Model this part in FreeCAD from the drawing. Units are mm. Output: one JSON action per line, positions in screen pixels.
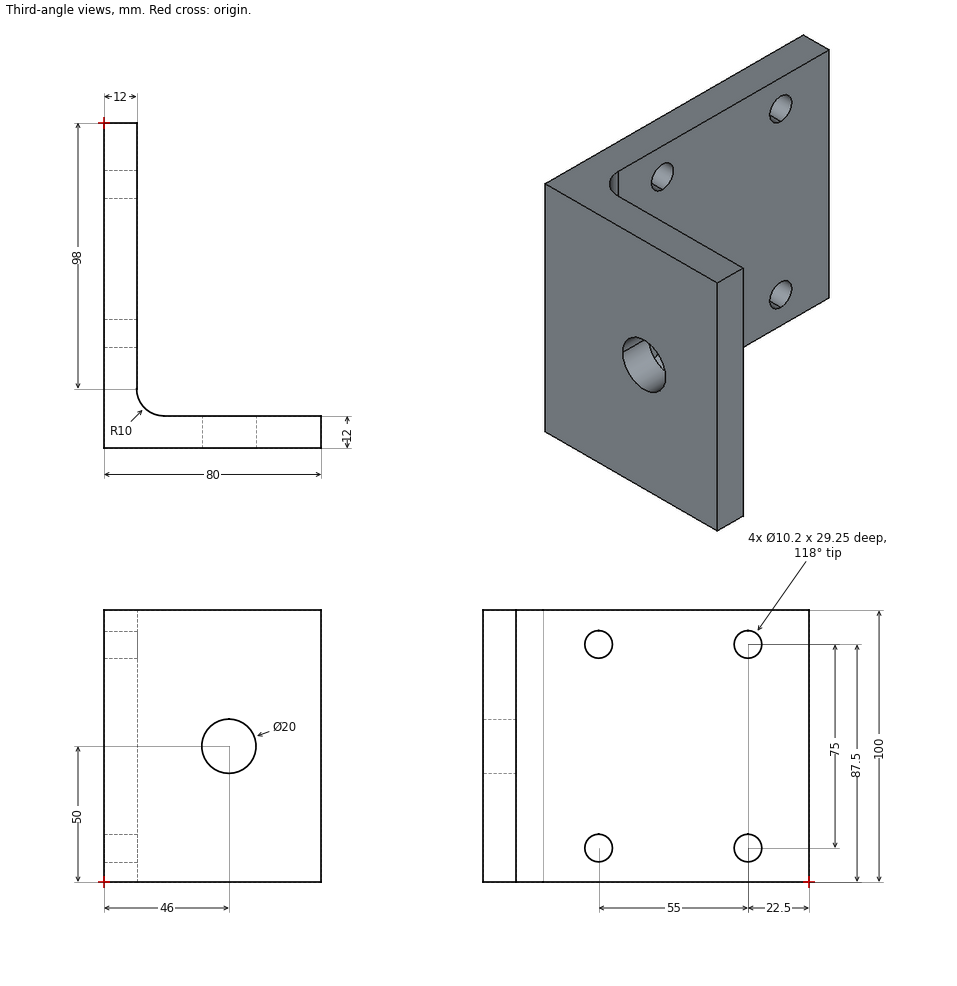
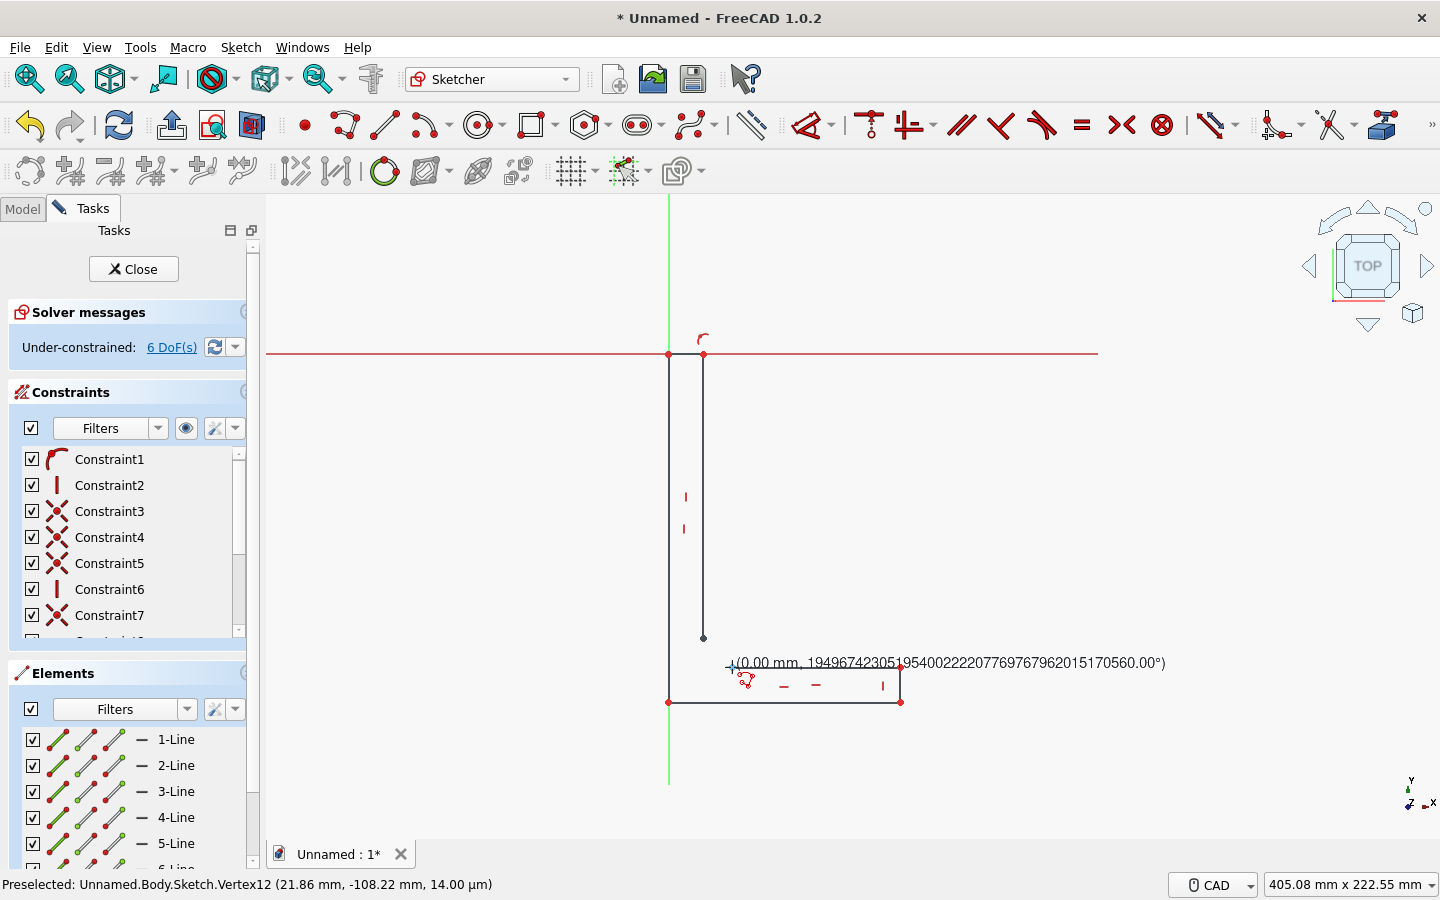
{"action": "left_click", "coordinate": [452, 126]}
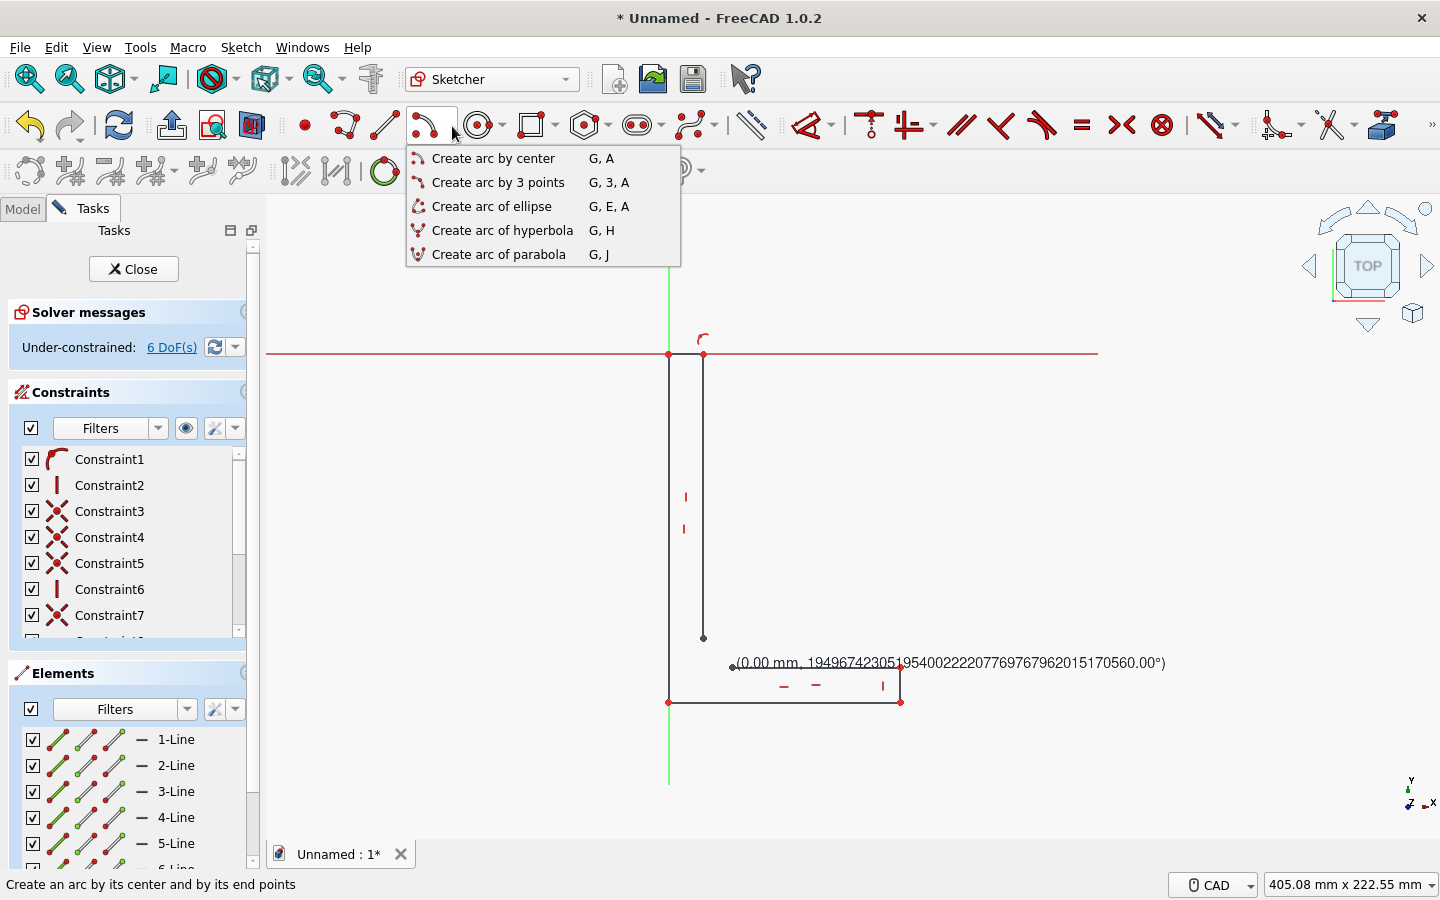
{"action": "left_click", "coordinate": [544, 182]}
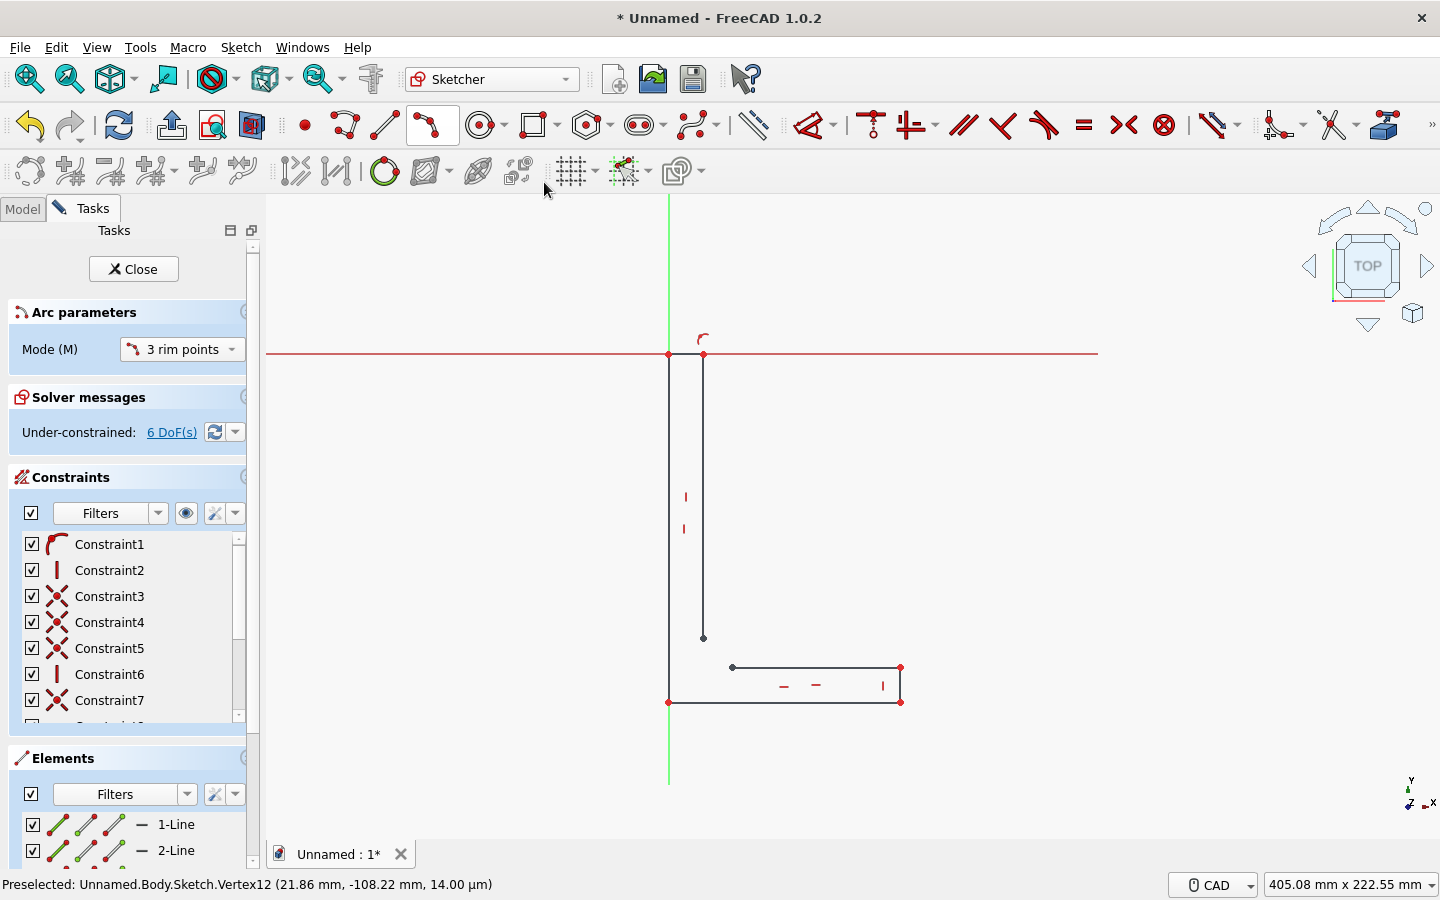
{"action": "left_click", "coordinate": [732, 668]}
{"action": "left_click", "coordinate": [703, 639]}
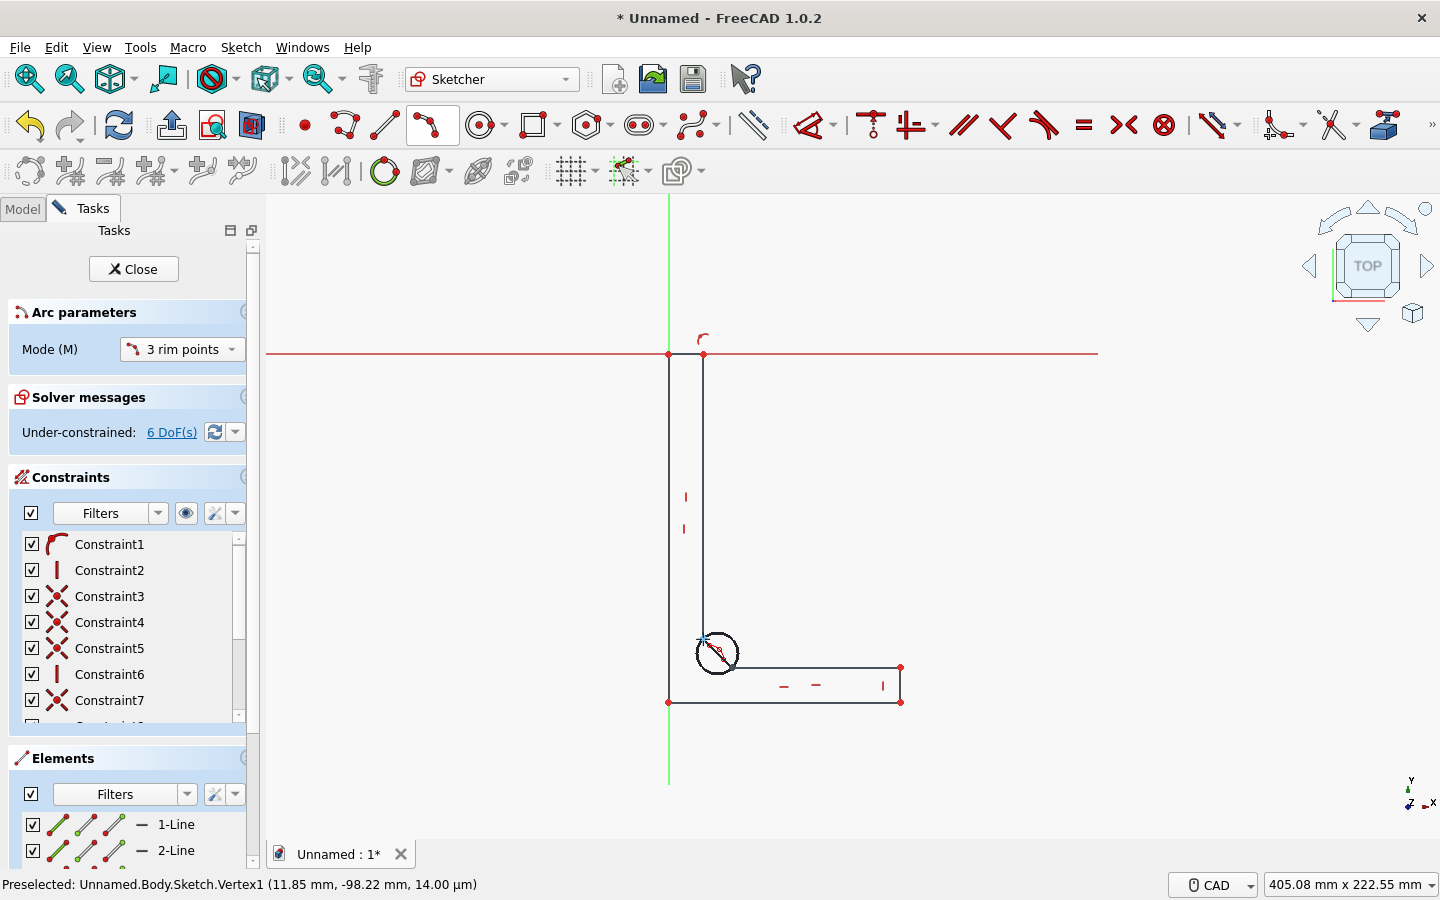
{"action": "scroll", "coordinate": [712, 659], "scroll_direction": "up", "scroll_amount": 4}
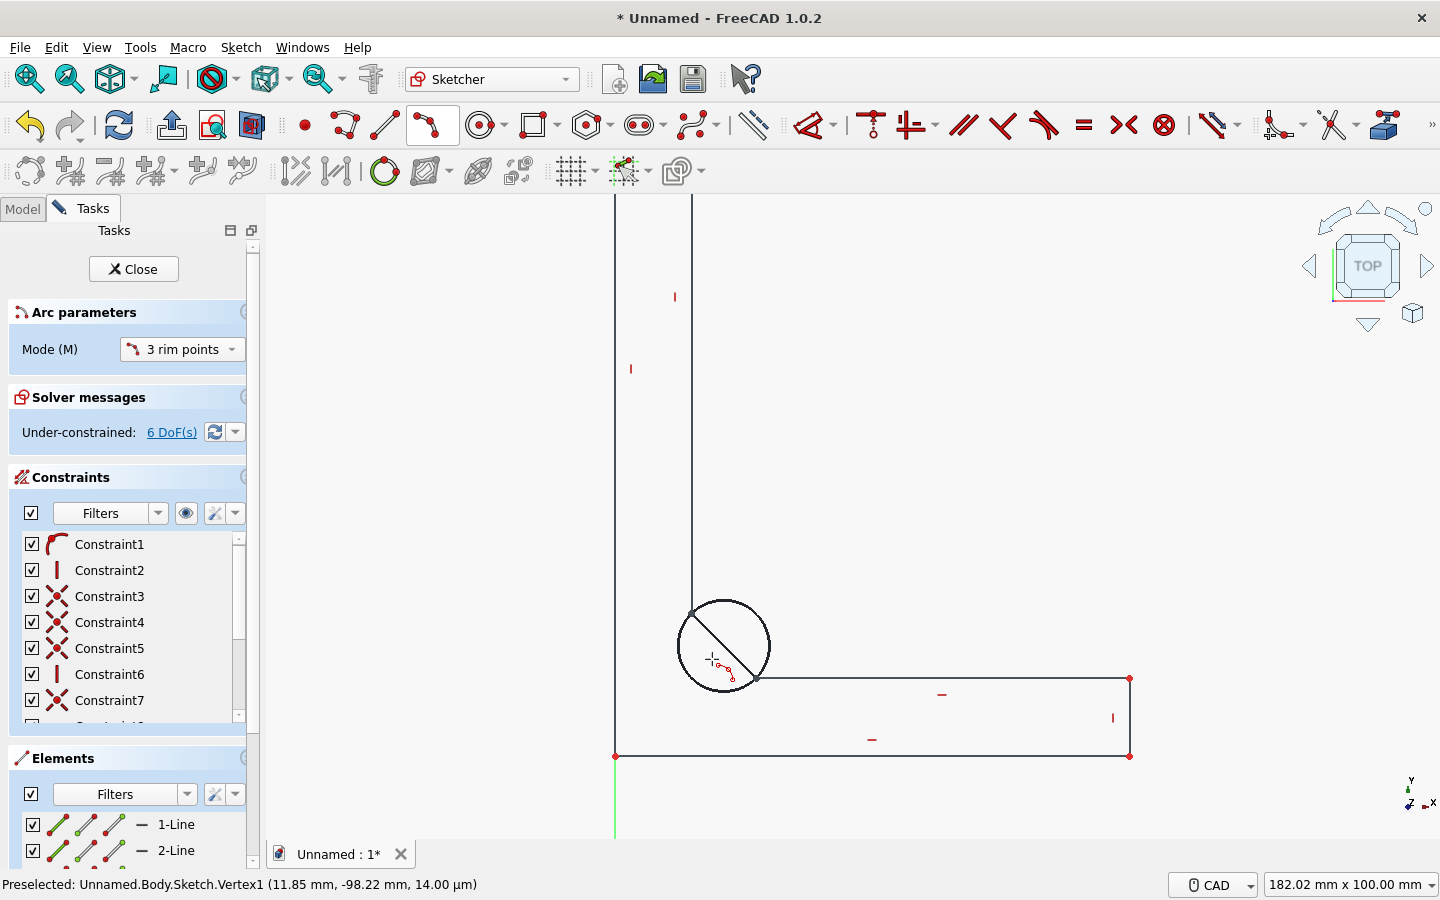
{"action": "left_click", "coordinate": [711, 658]}
{"action": "key", "text": "Escape"}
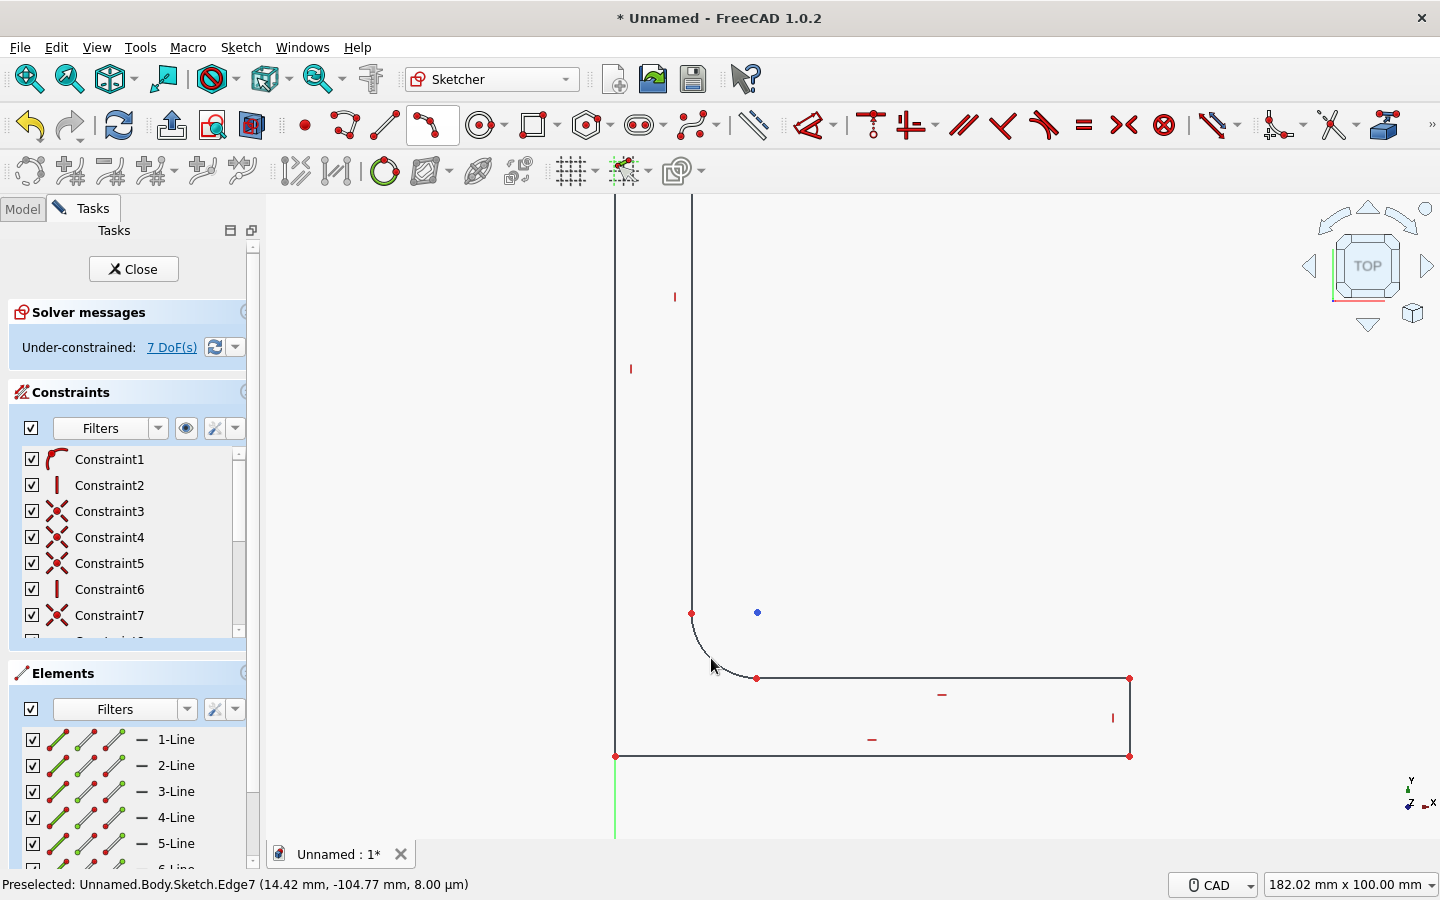
{"action": "left_click", "coordinate": [692, 424]}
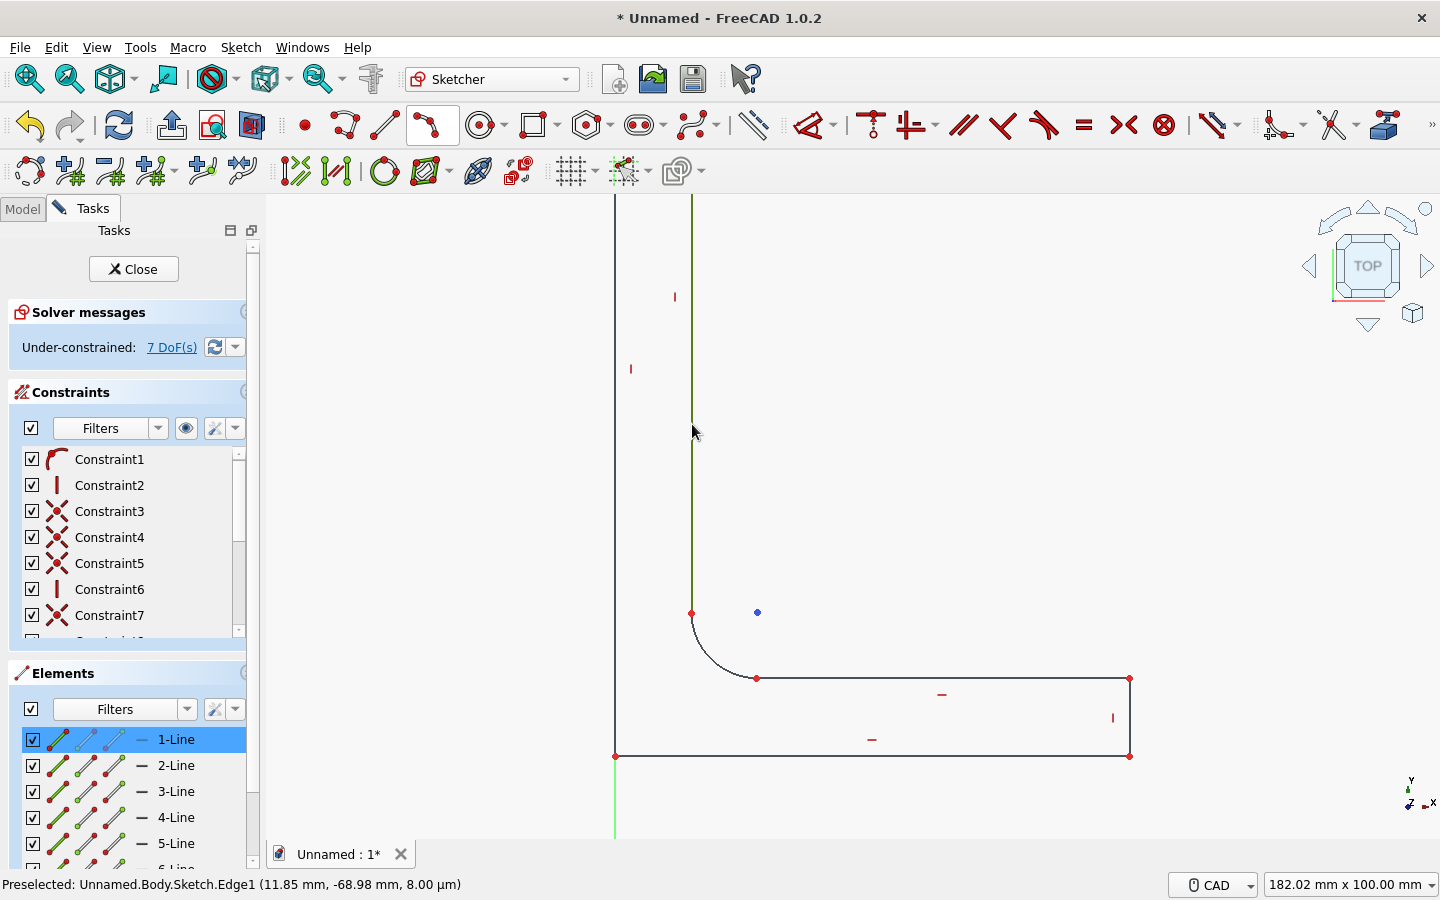
{"action": "left_click", "coordinate": [699, 643]}